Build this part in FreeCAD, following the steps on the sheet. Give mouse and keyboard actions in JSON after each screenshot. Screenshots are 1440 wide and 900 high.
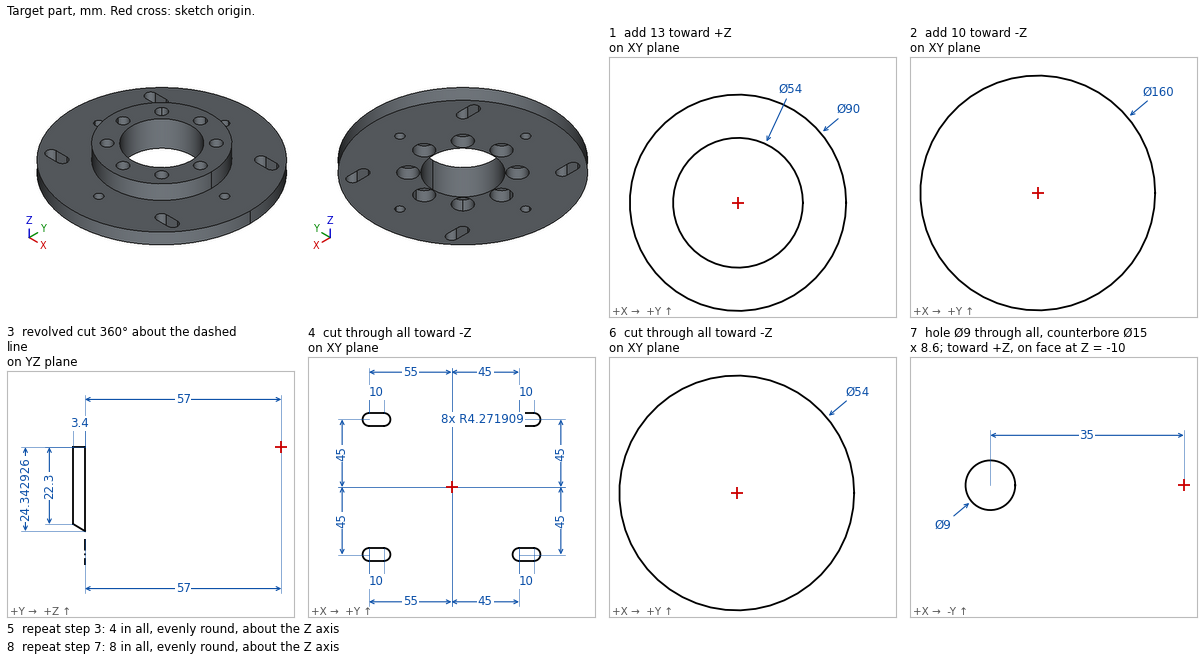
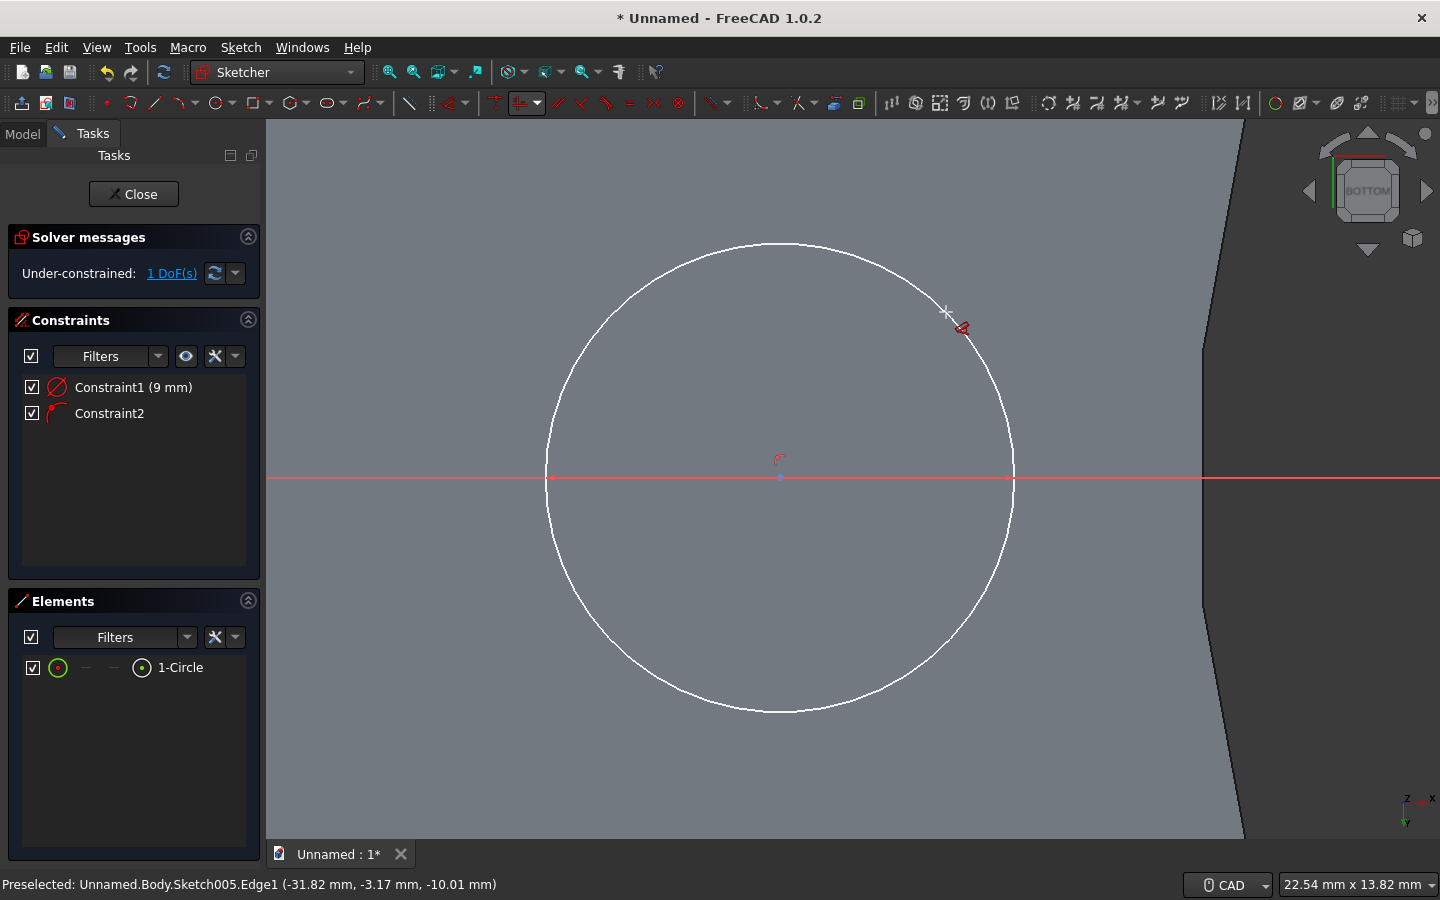
{"action": "left_click", "coordinate": [780, 478]}
{"action": "left_click", "coordinate": [1028, 512]}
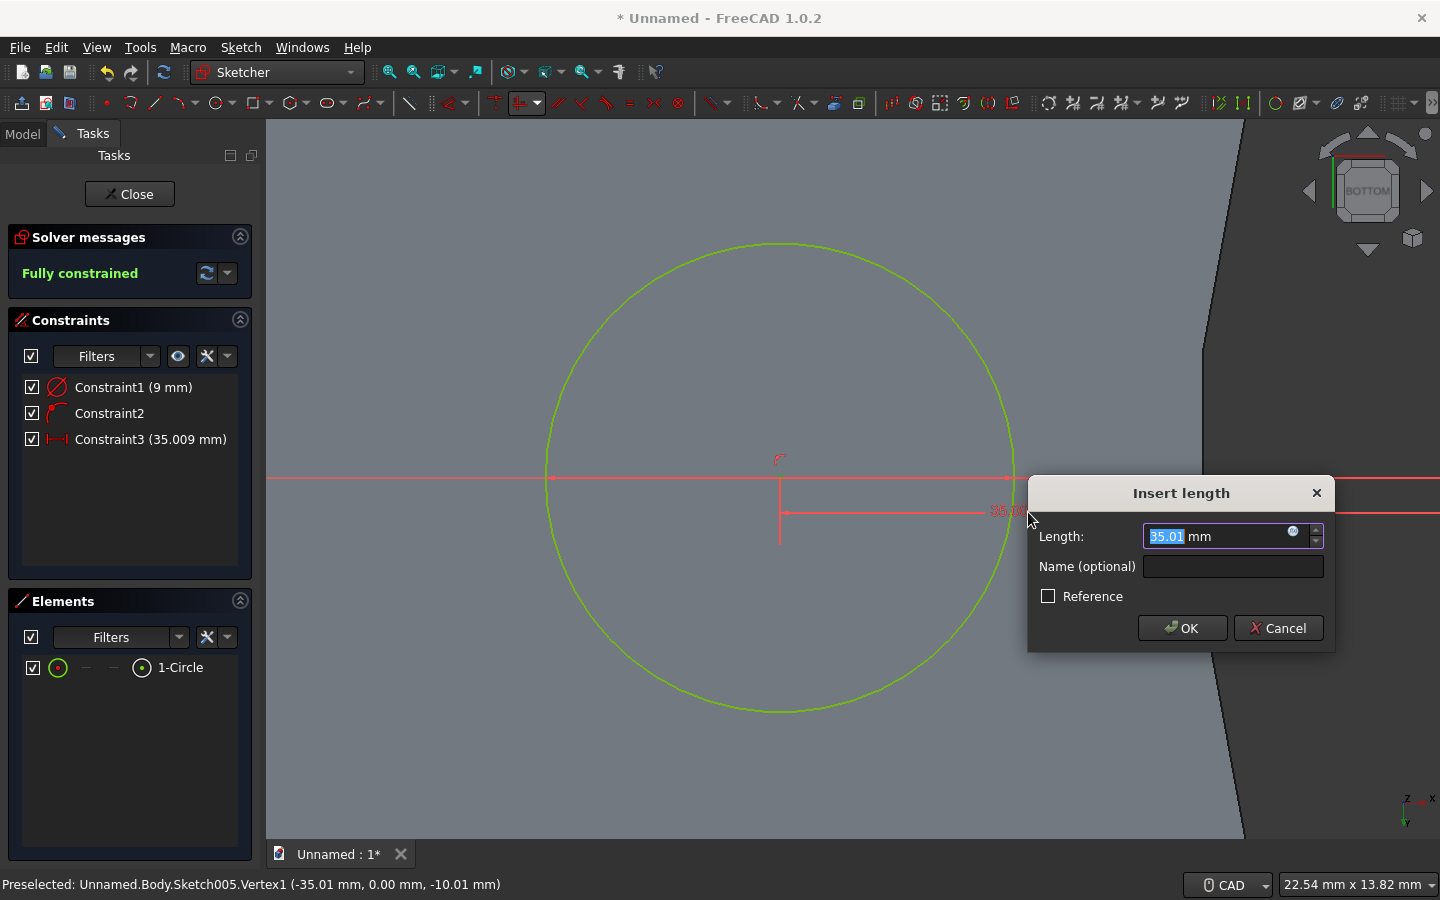
{"action": "type", "text": "35"}
{"action": "key", "text": "Return"}
{"action": "key", "text": "Escape"}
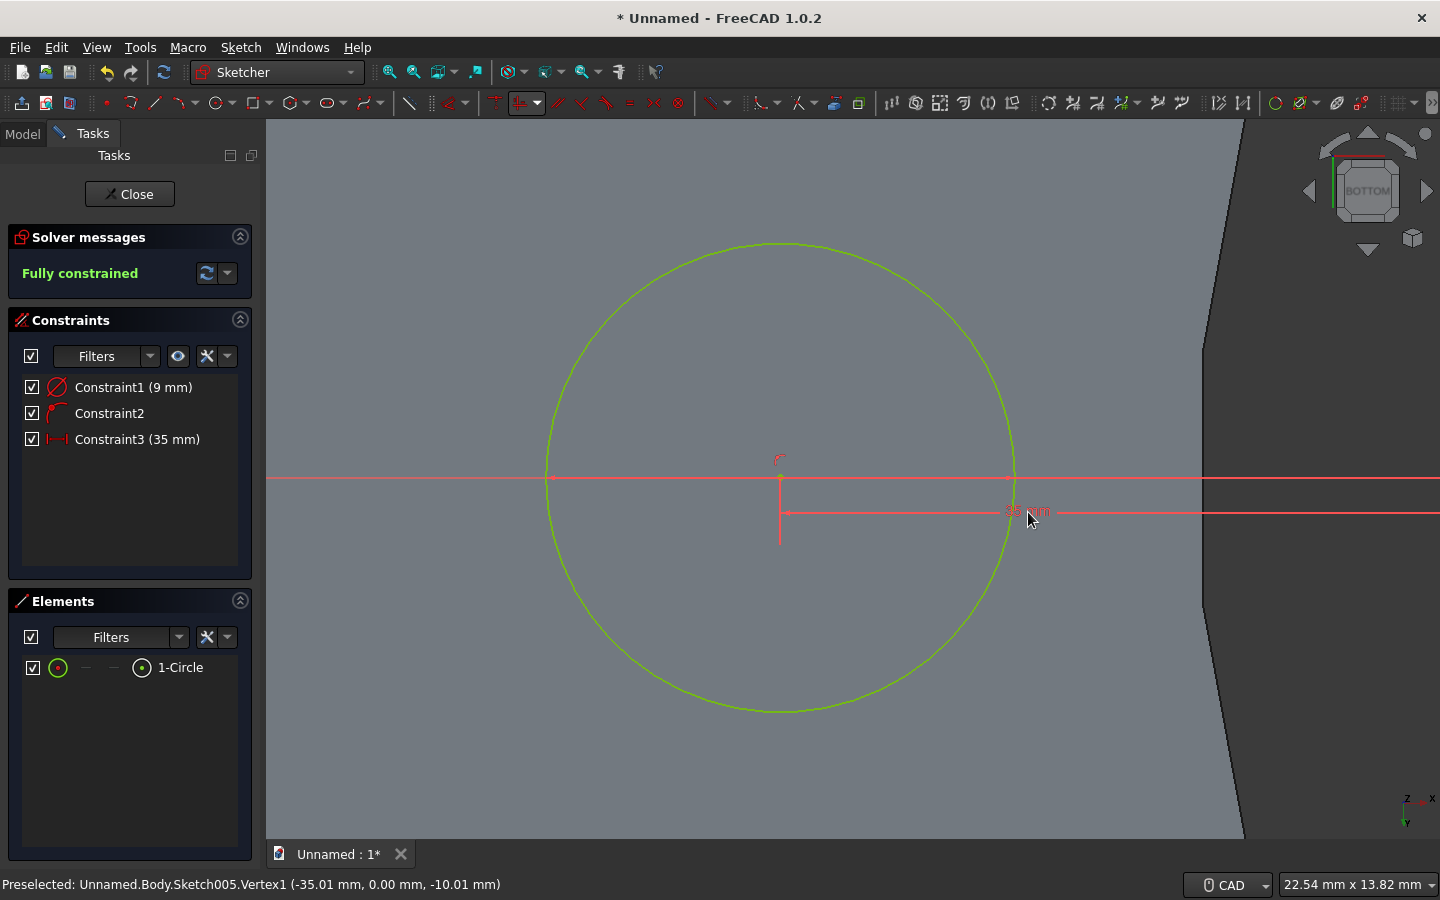
{"action": "left_click", "coordinate": [130, 194]}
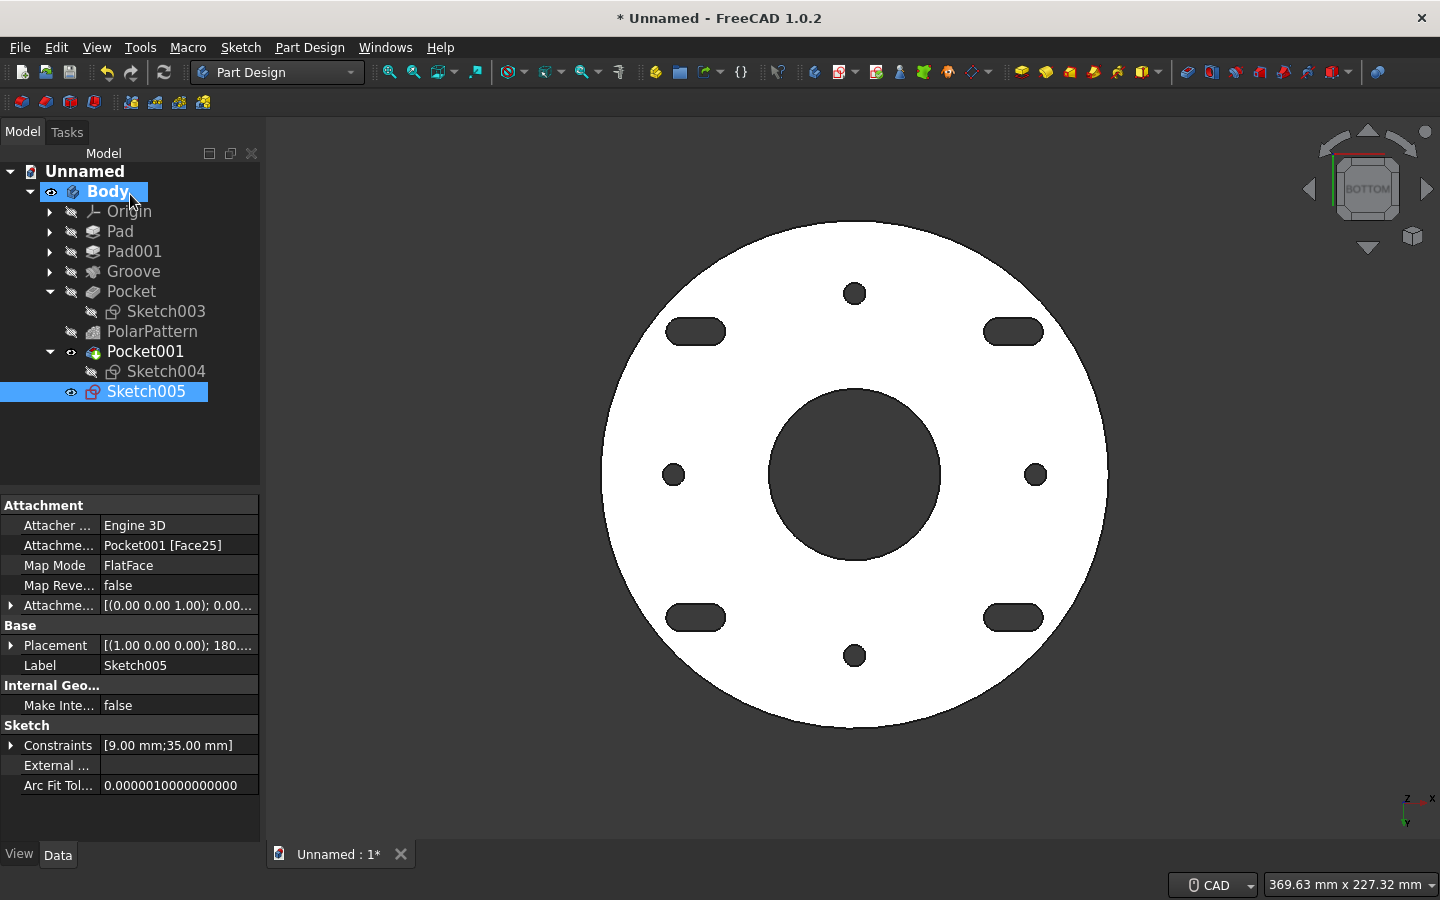
{"action": "left_click", "coordinate": [1212, 72]}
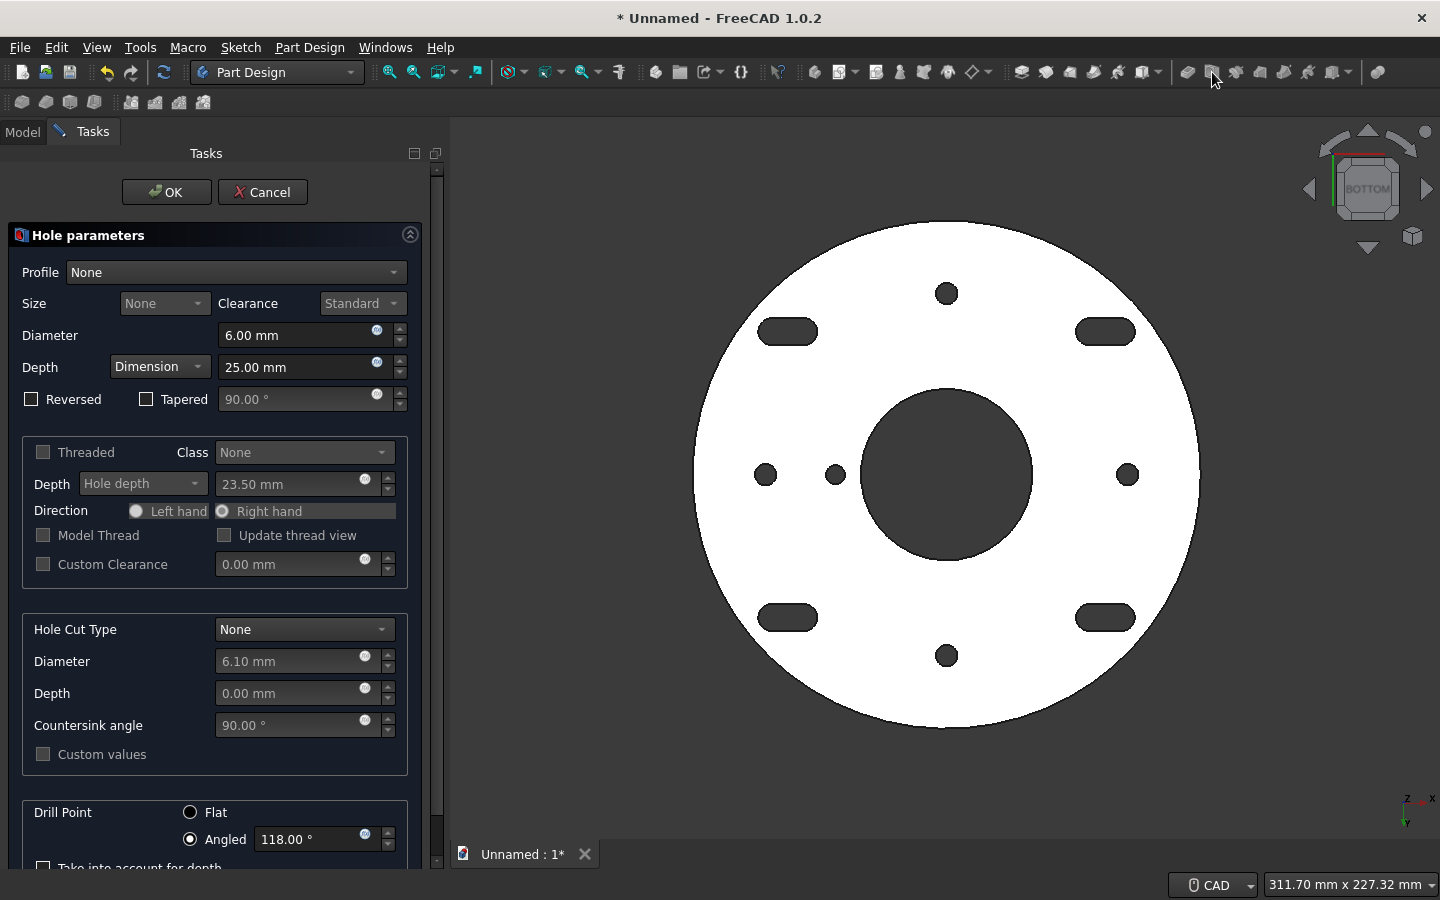
{"action": "triple_click", "coordinate": [305, 335]}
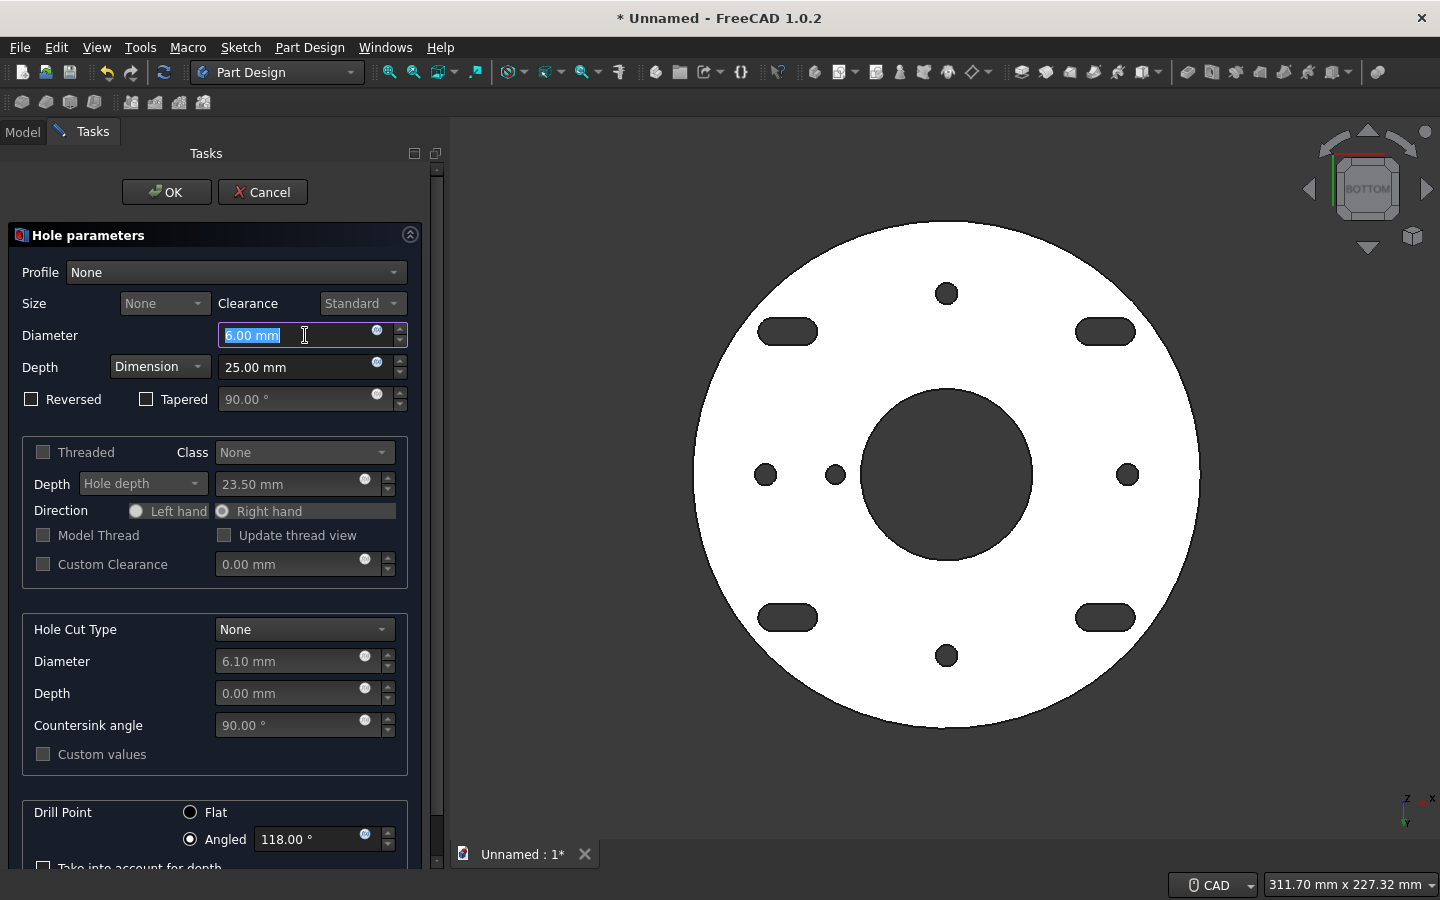
{"action": "type", "text": "9"}
{"action": "key", "text": "Tab"}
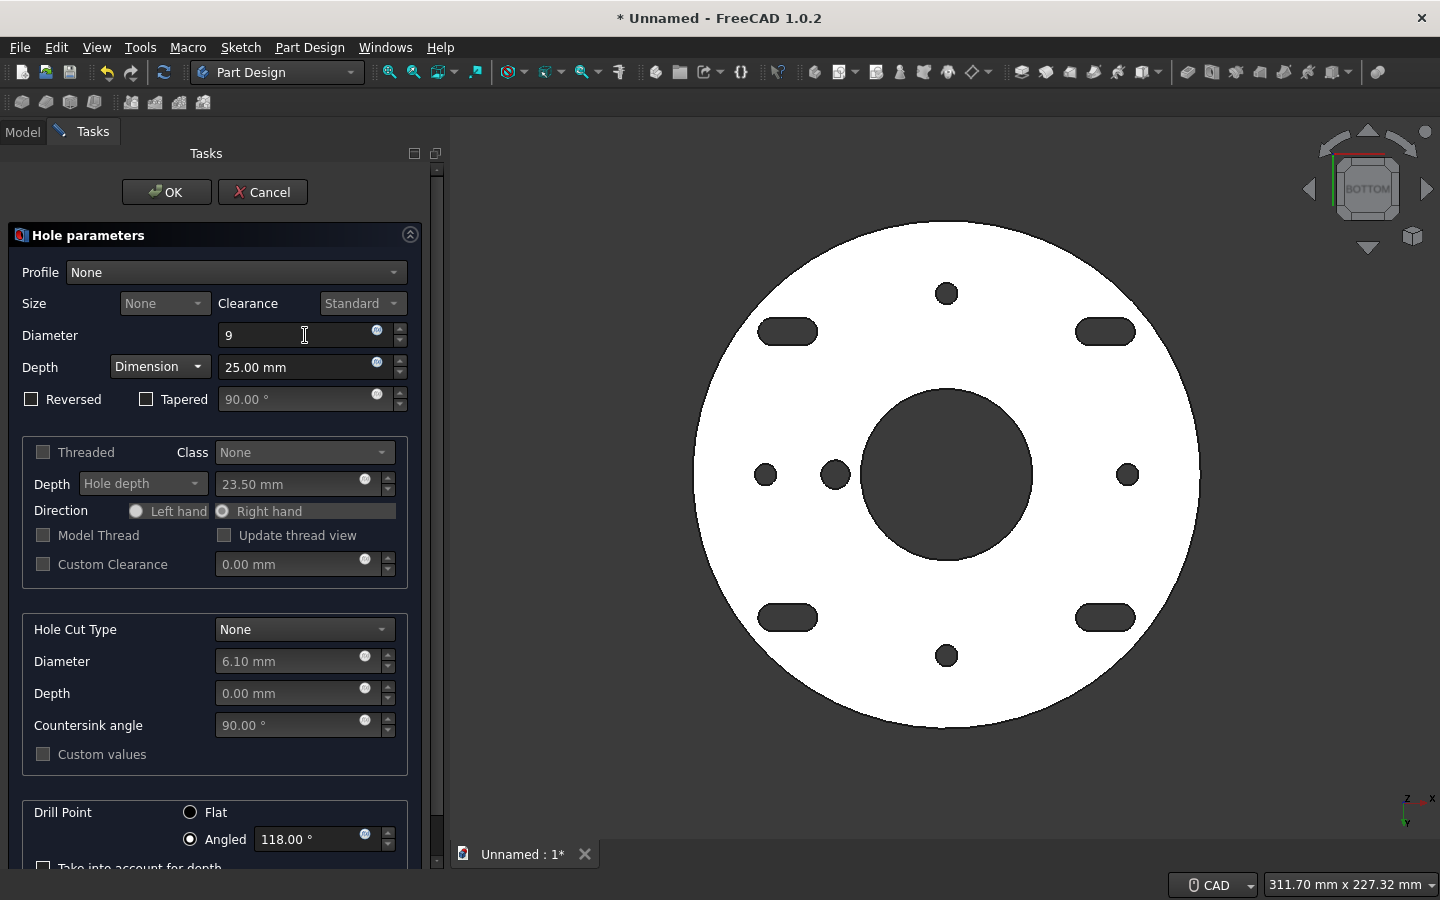
{"action": "left_click", "coordinate": [161, 366]}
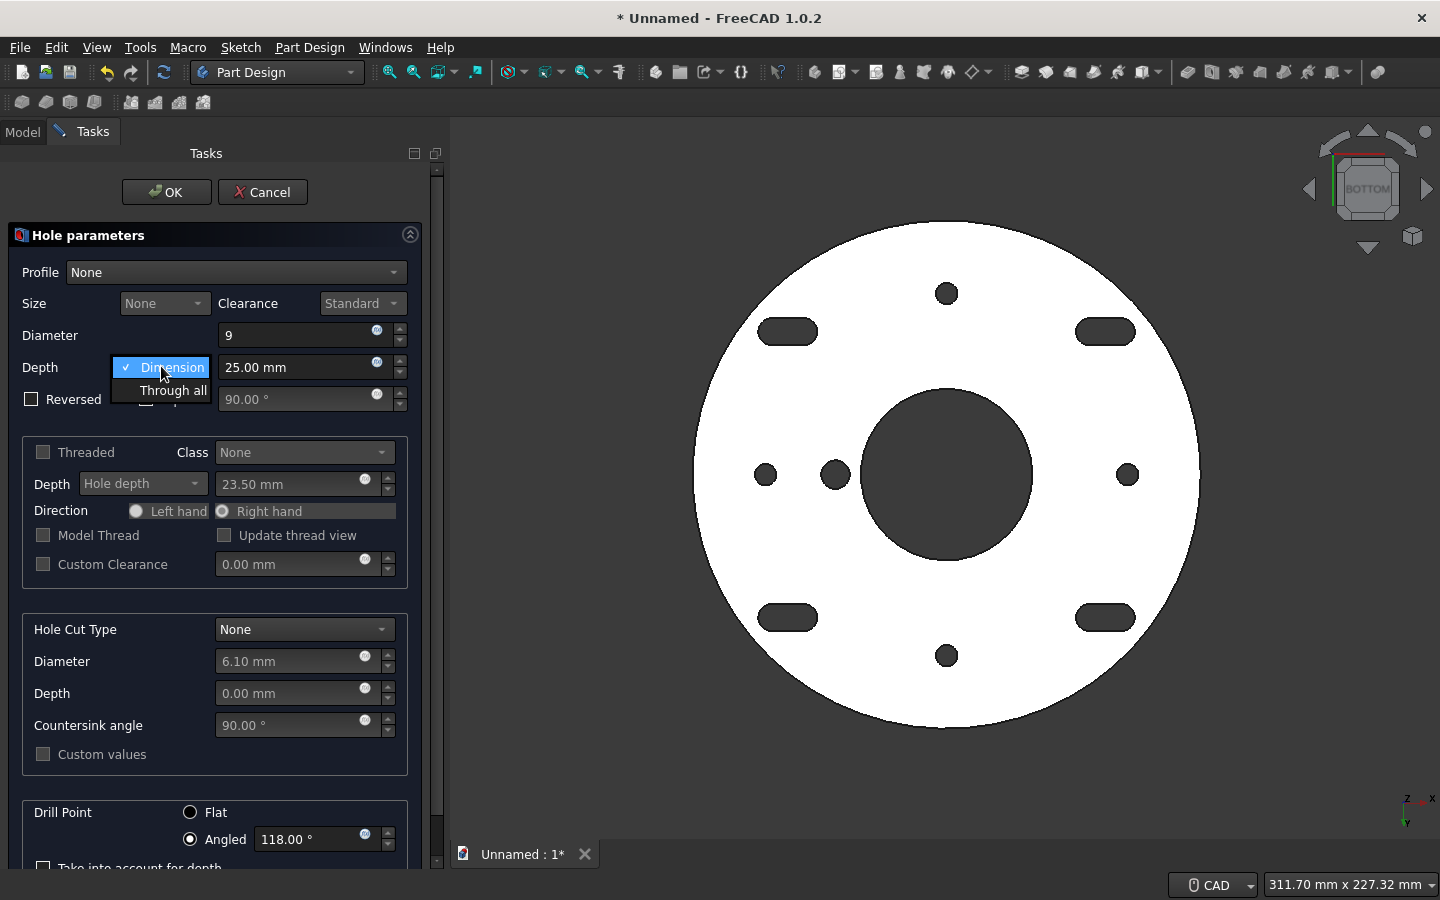
{"action": "left_click", "coordinate": [160, 390]}